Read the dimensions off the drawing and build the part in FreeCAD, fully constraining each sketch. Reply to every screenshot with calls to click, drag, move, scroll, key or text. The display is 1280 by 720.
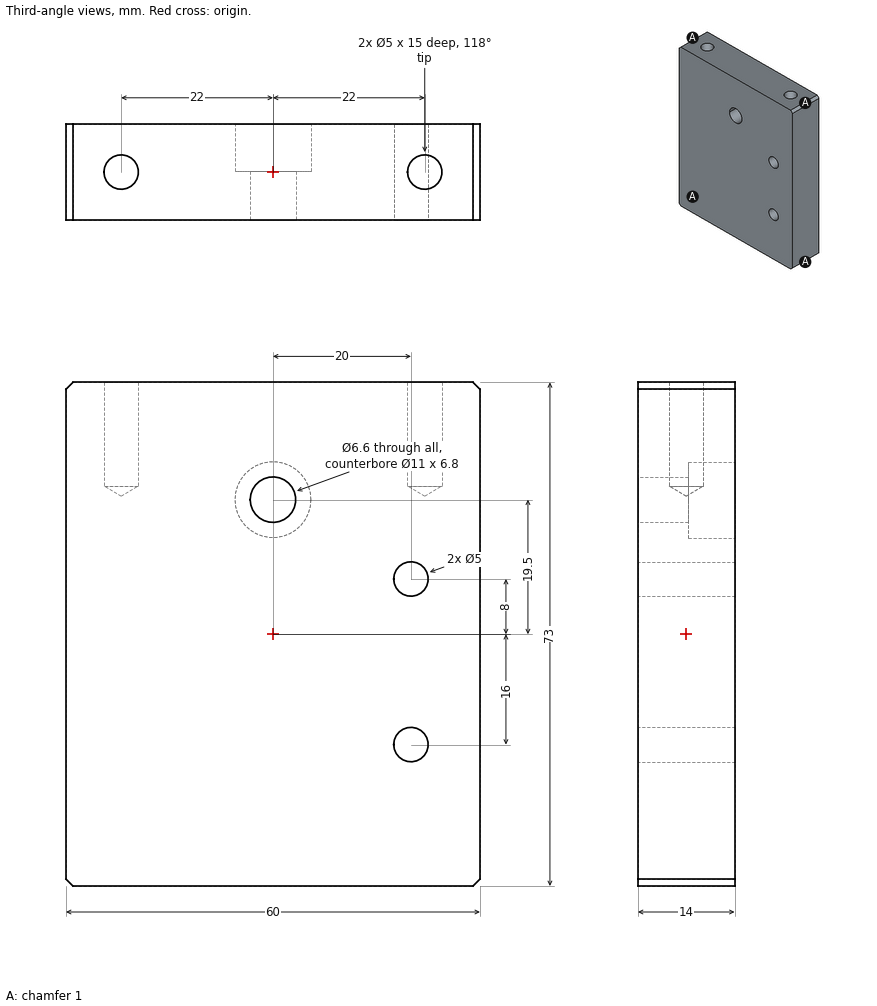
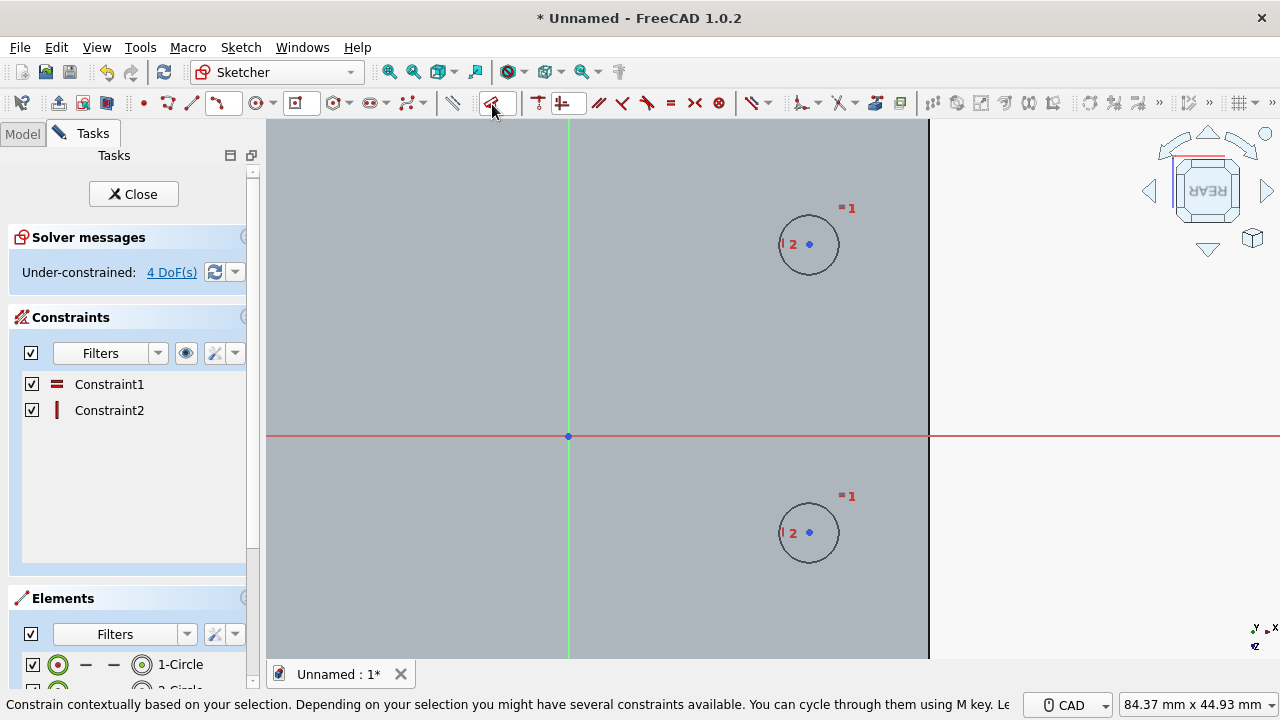
click(830, 512)
click(853, 489)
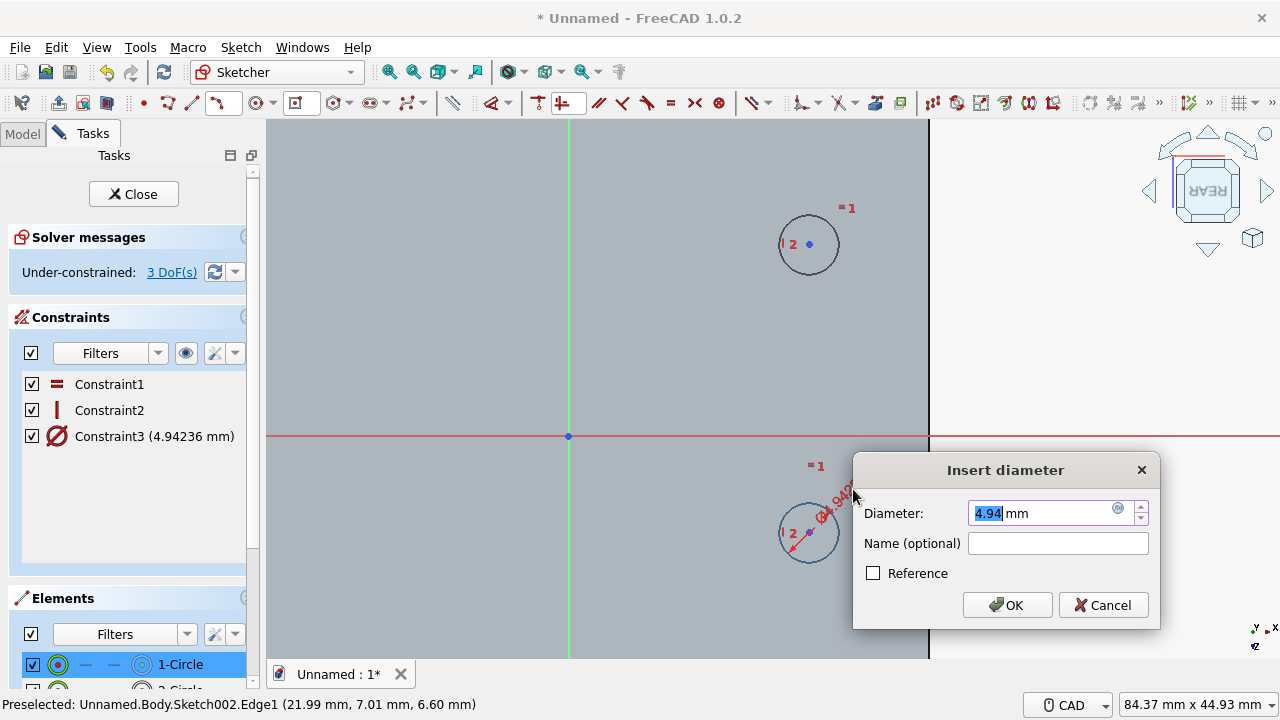
text(5)
key(Return)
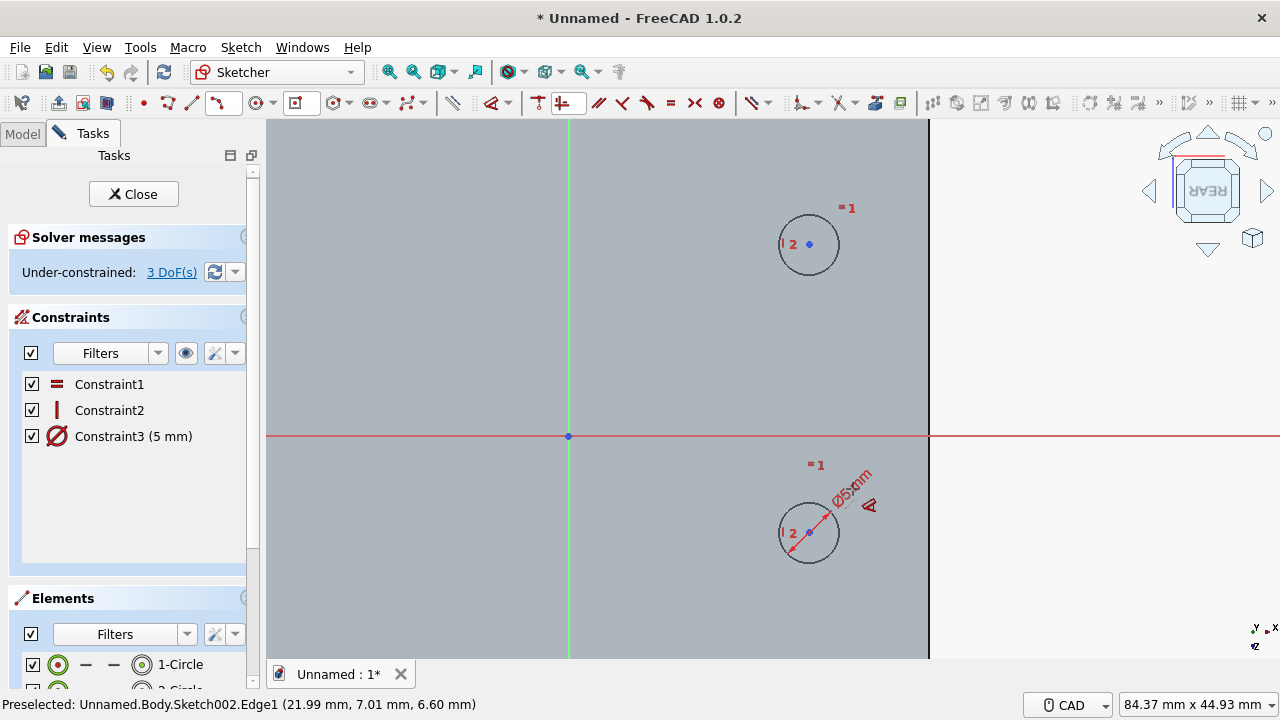
click(809, 533)
click(535, 485)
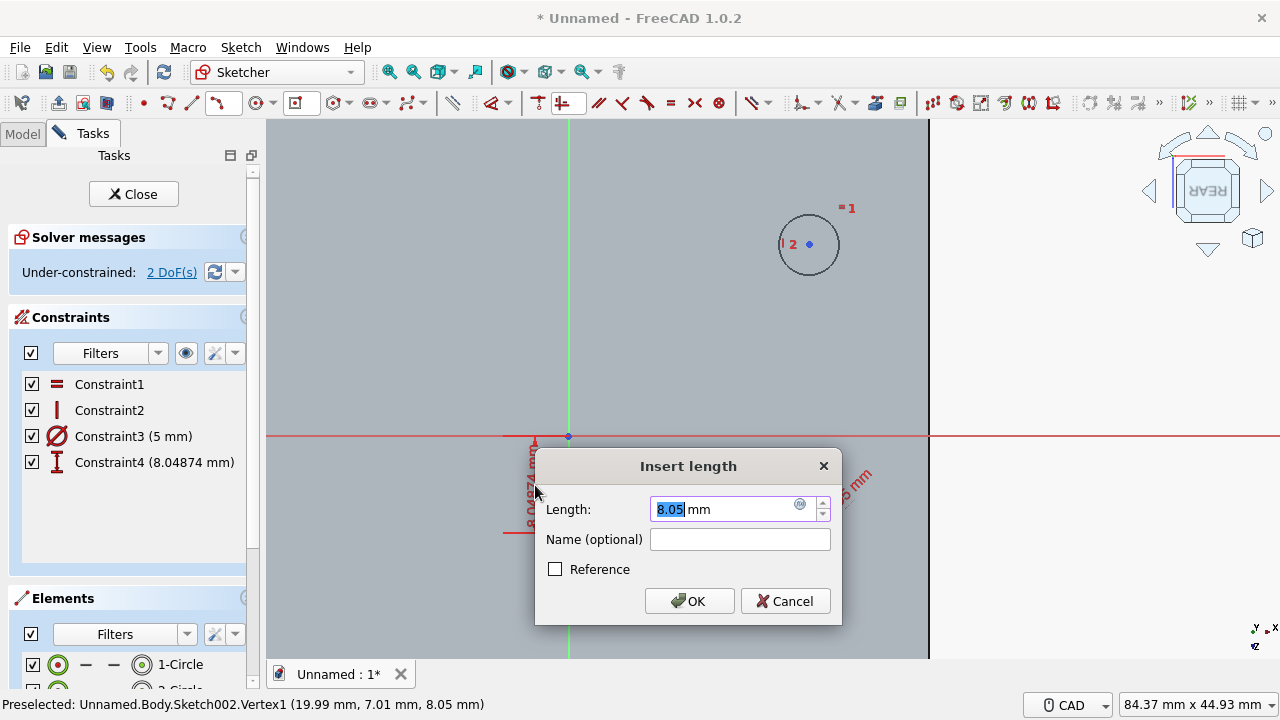
text(8)
key(Return)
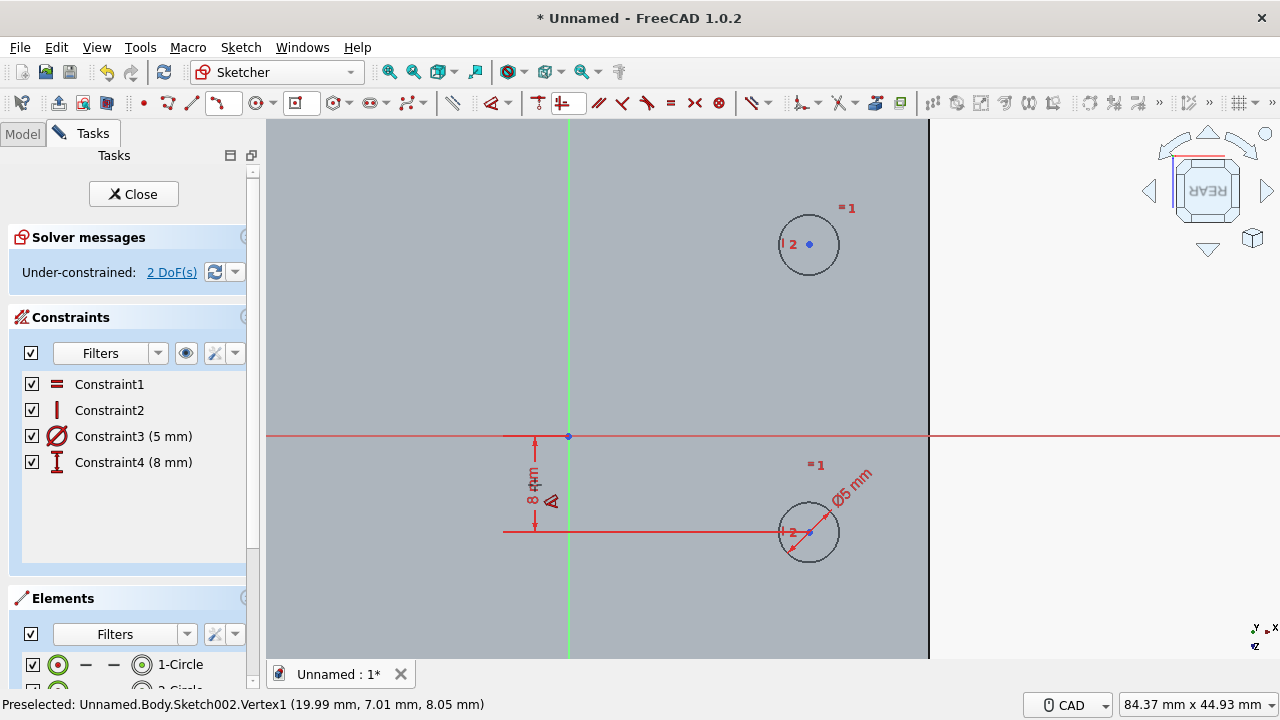
click(809, 532)
click(689, 566)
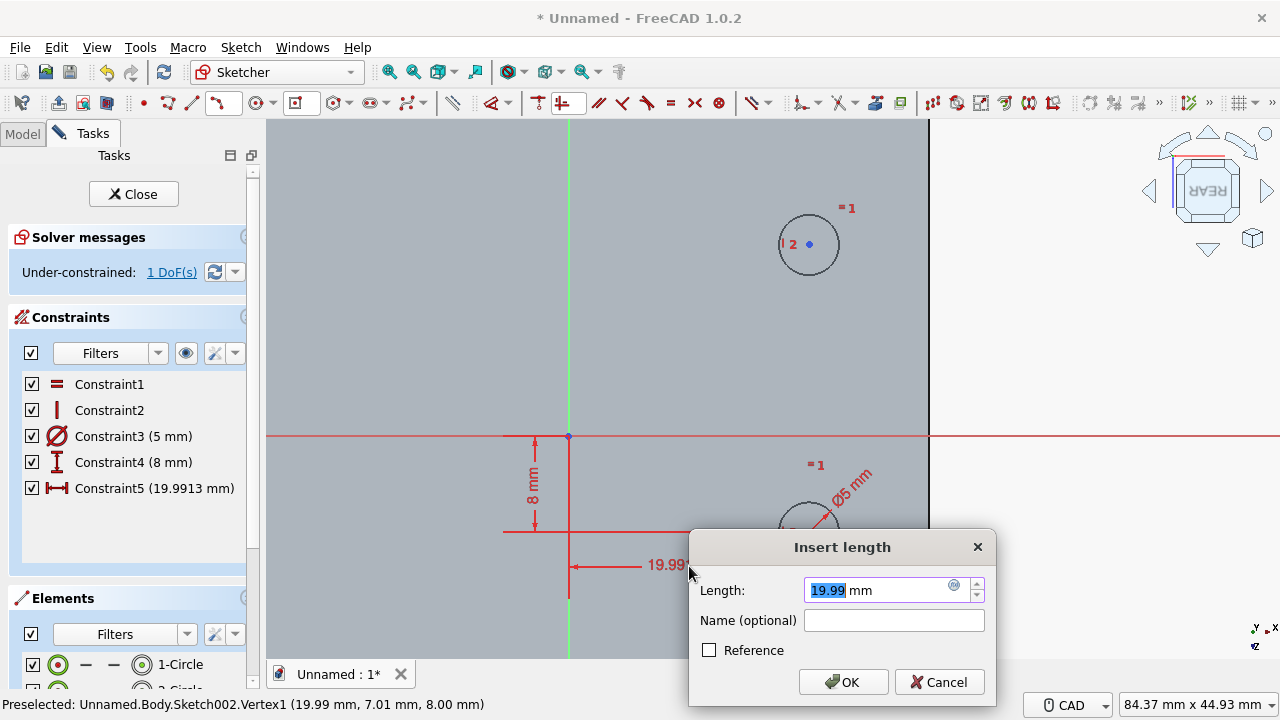
text(20)
key(Return)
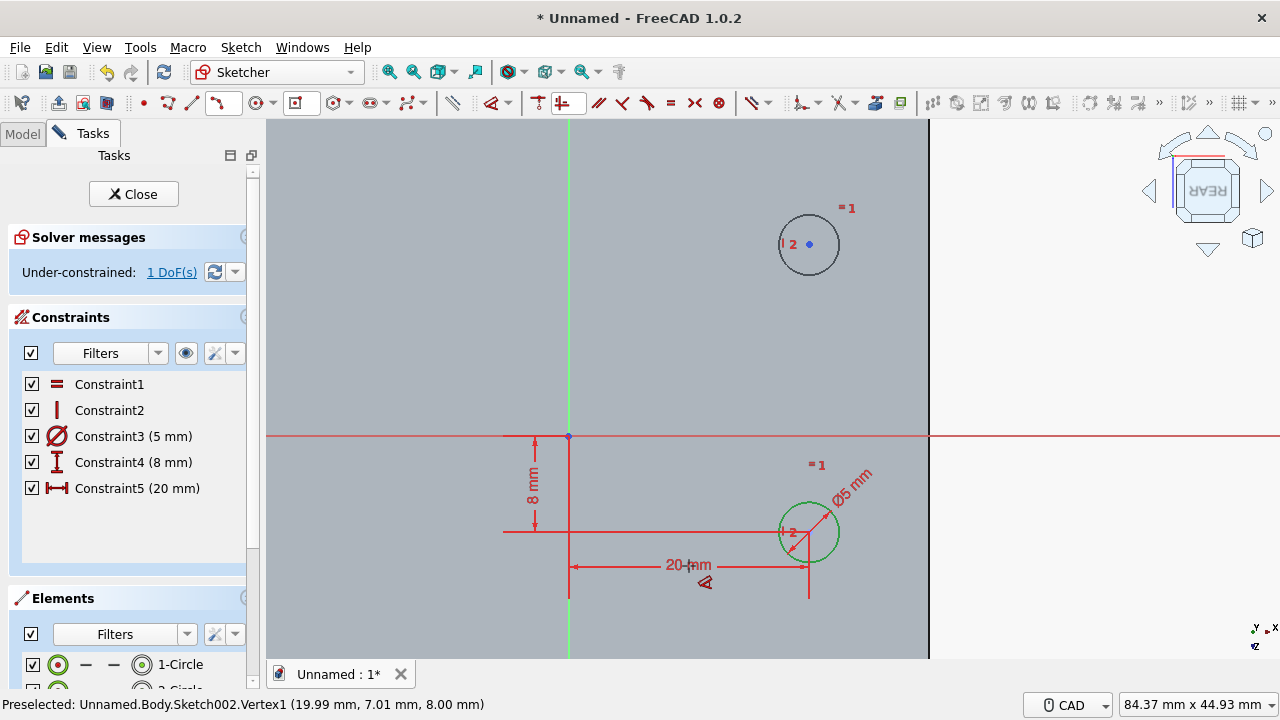
click(809, 245)
click(535, 341)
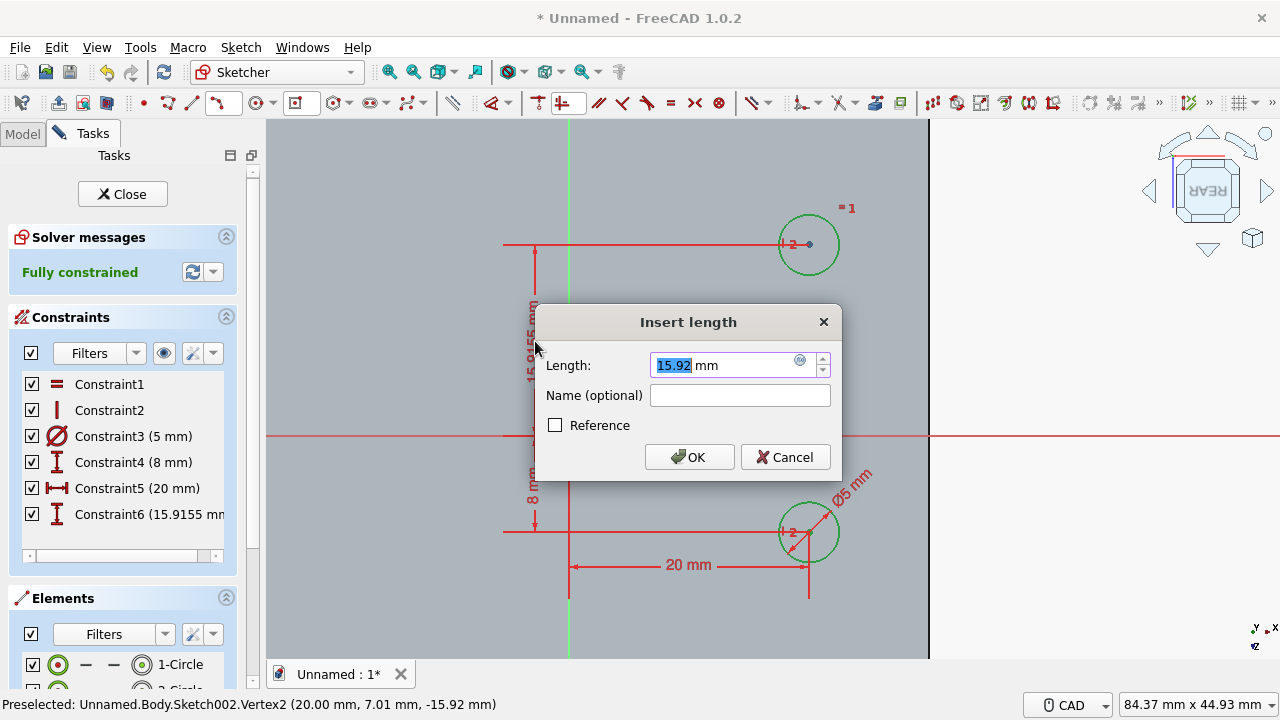
text(16)
key(Return)
key(Escape)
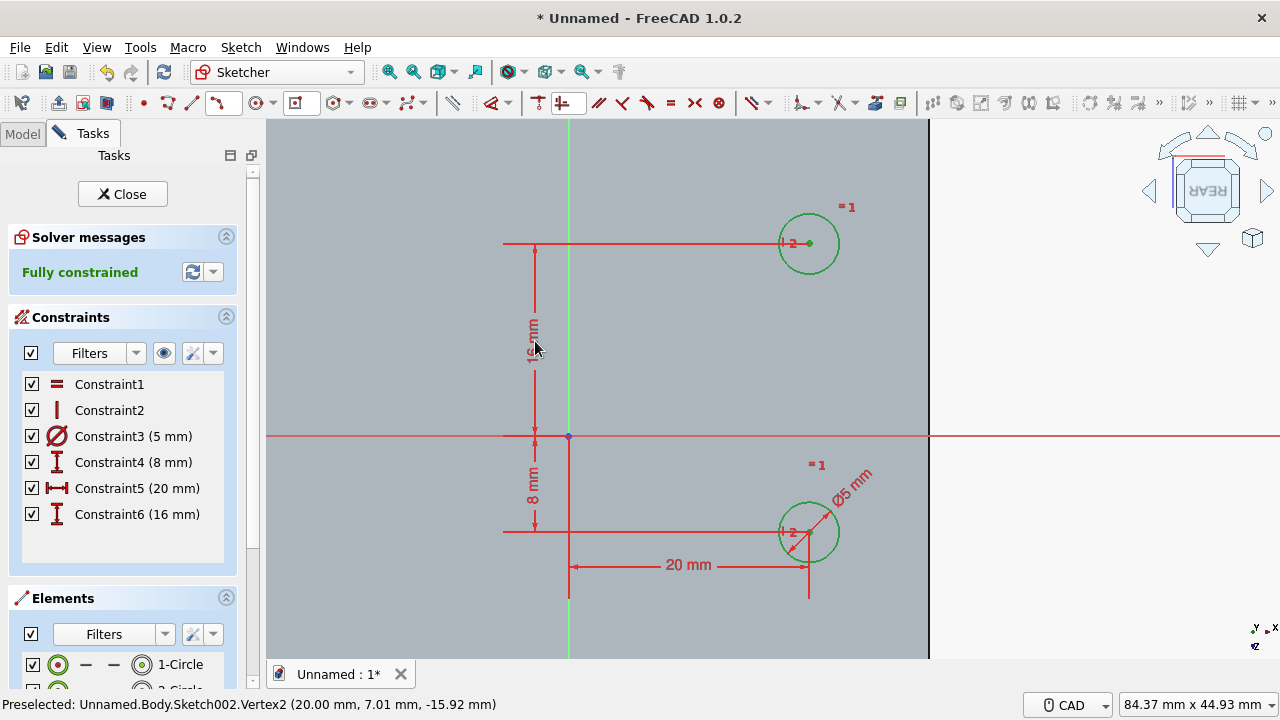
click(123, 194)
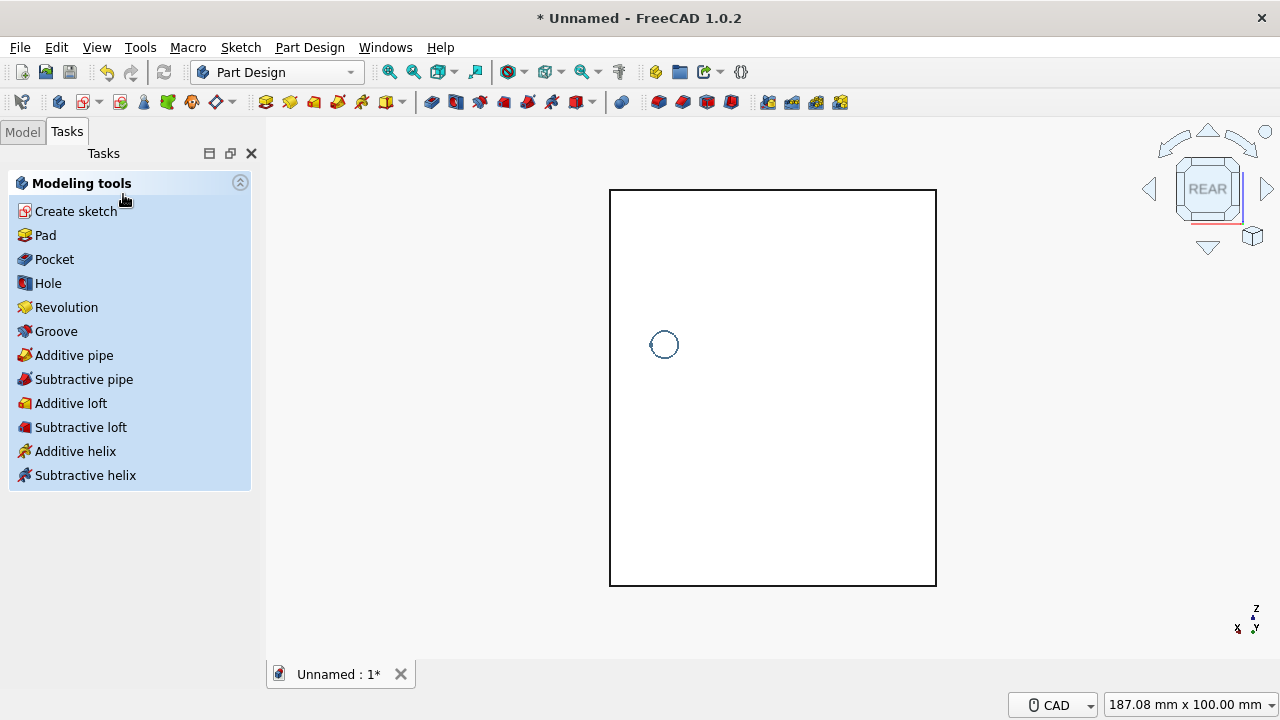
click(432, 102)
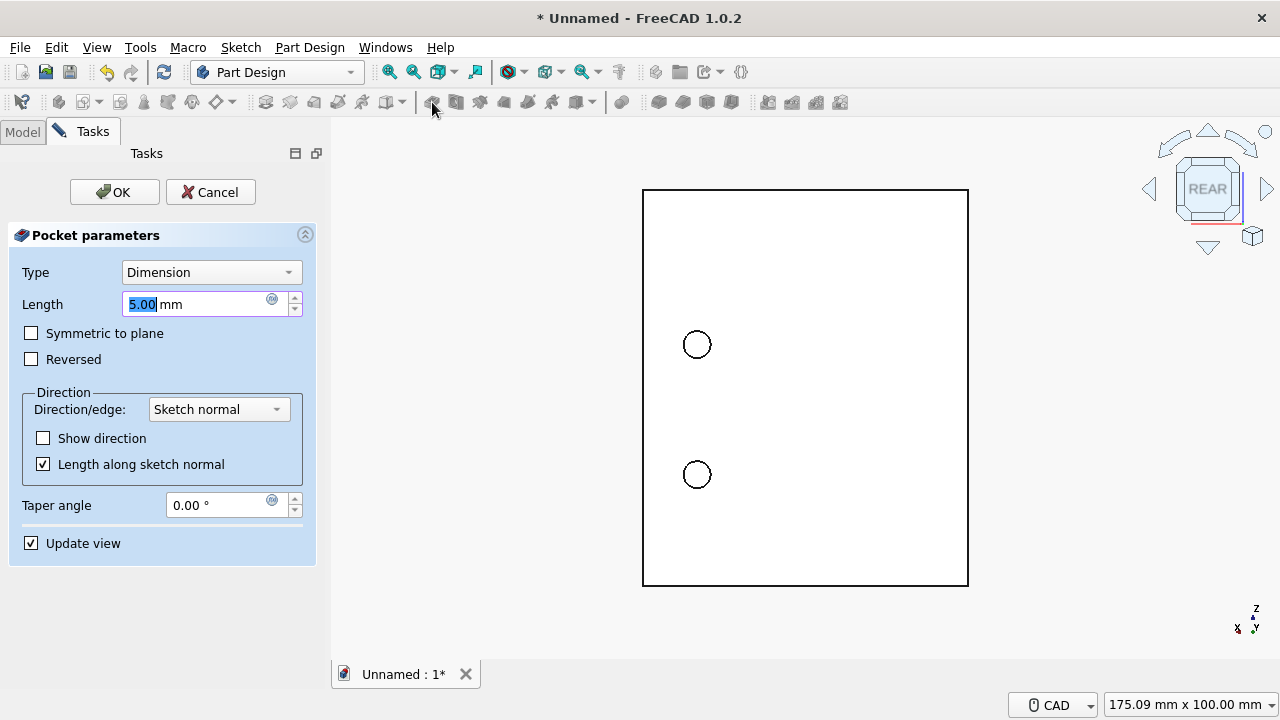
click(212, 272)